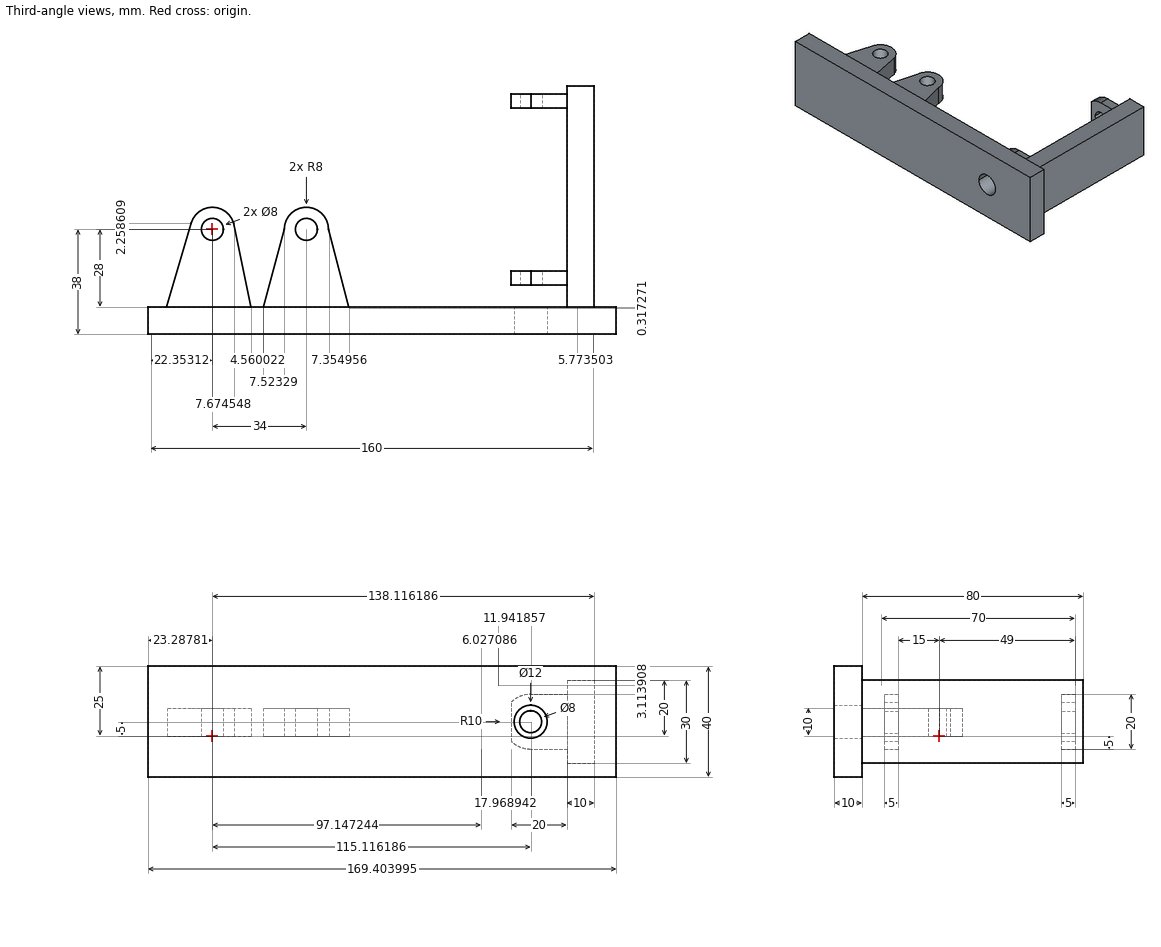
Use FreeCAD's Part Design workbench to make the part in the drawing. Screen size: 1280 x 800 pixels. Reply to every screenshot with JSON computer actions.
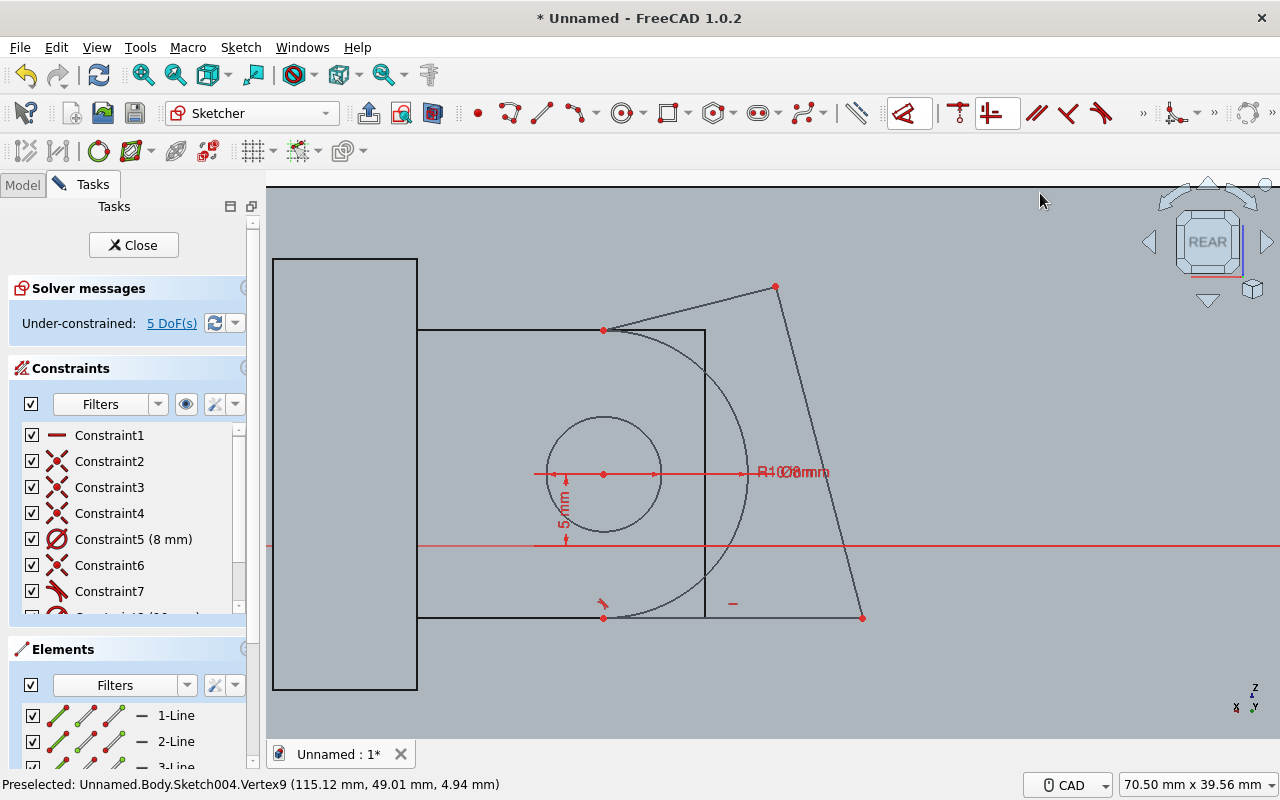
{"action": "left_click", "coordinate": [682, 618]}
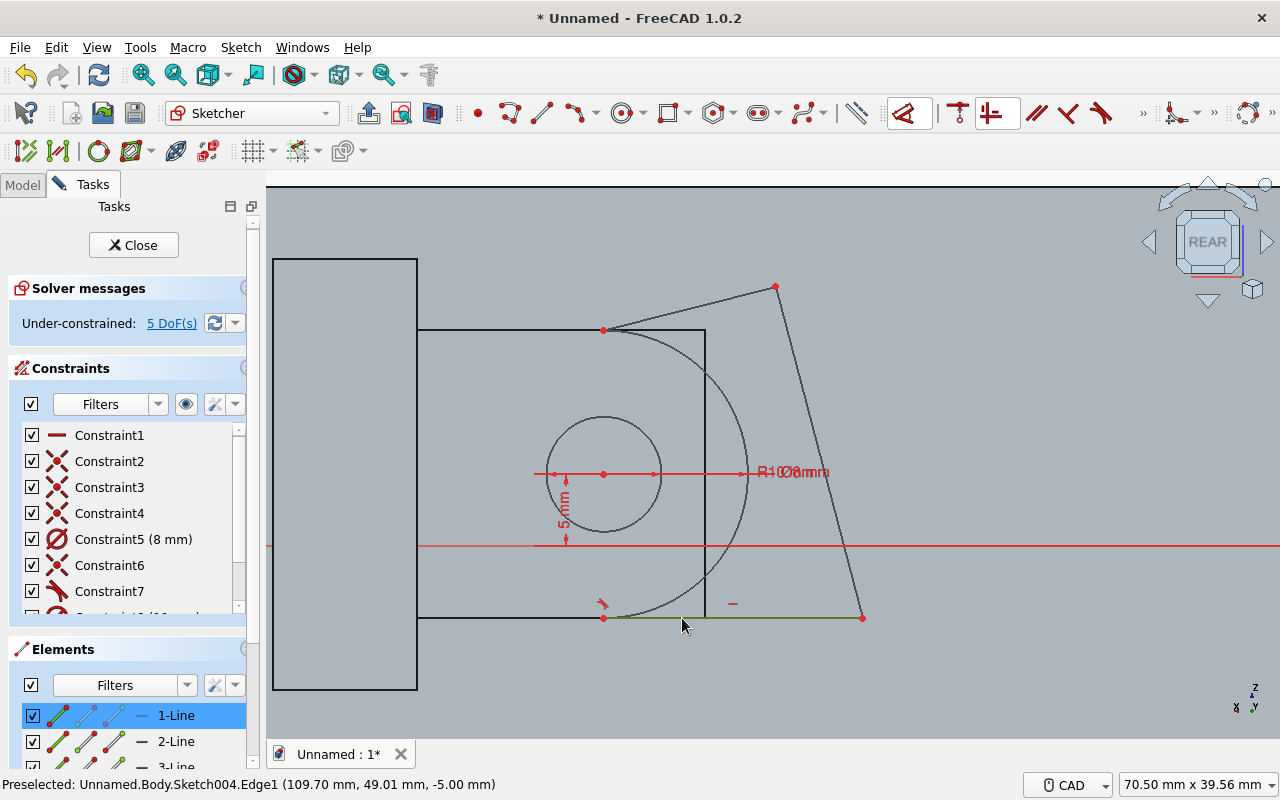
{"action": "left_click", "coordinate": [926, 114]}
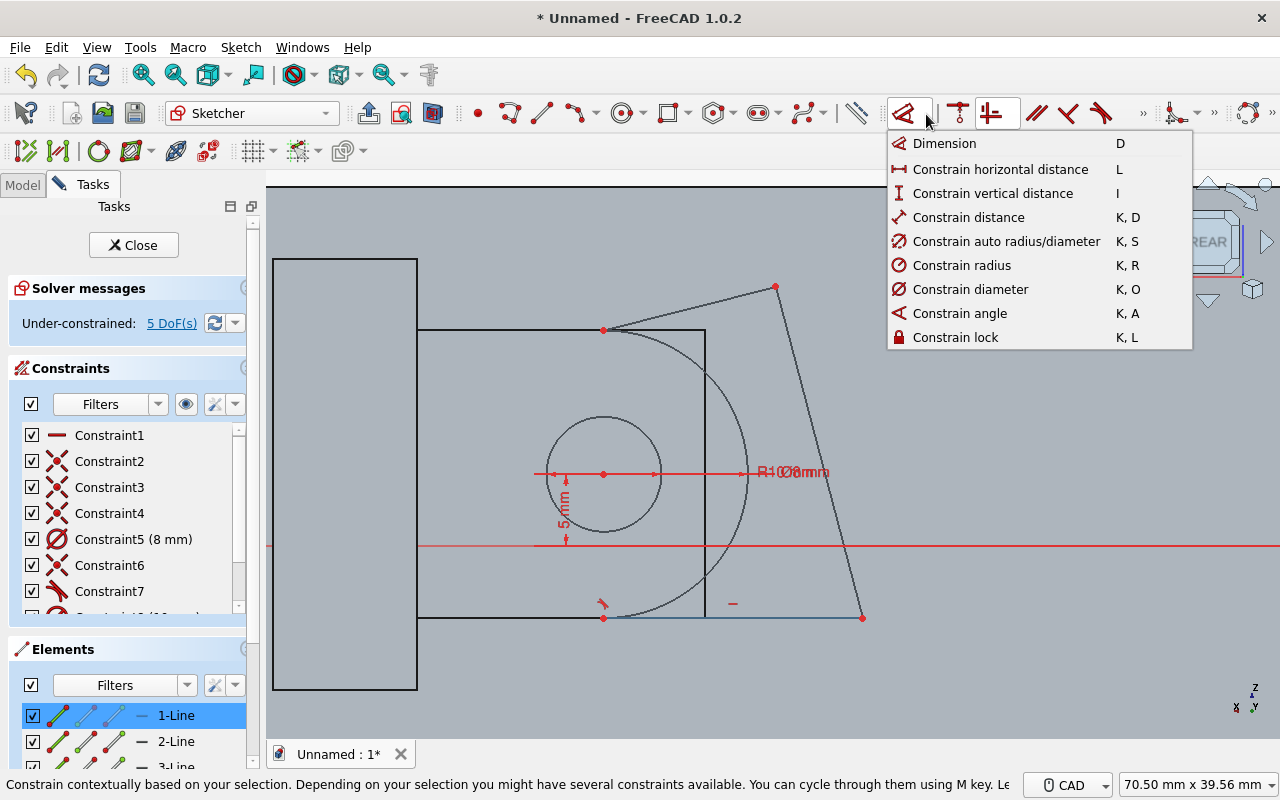
{"action": "left_click", "coordinate": [1040, 169]}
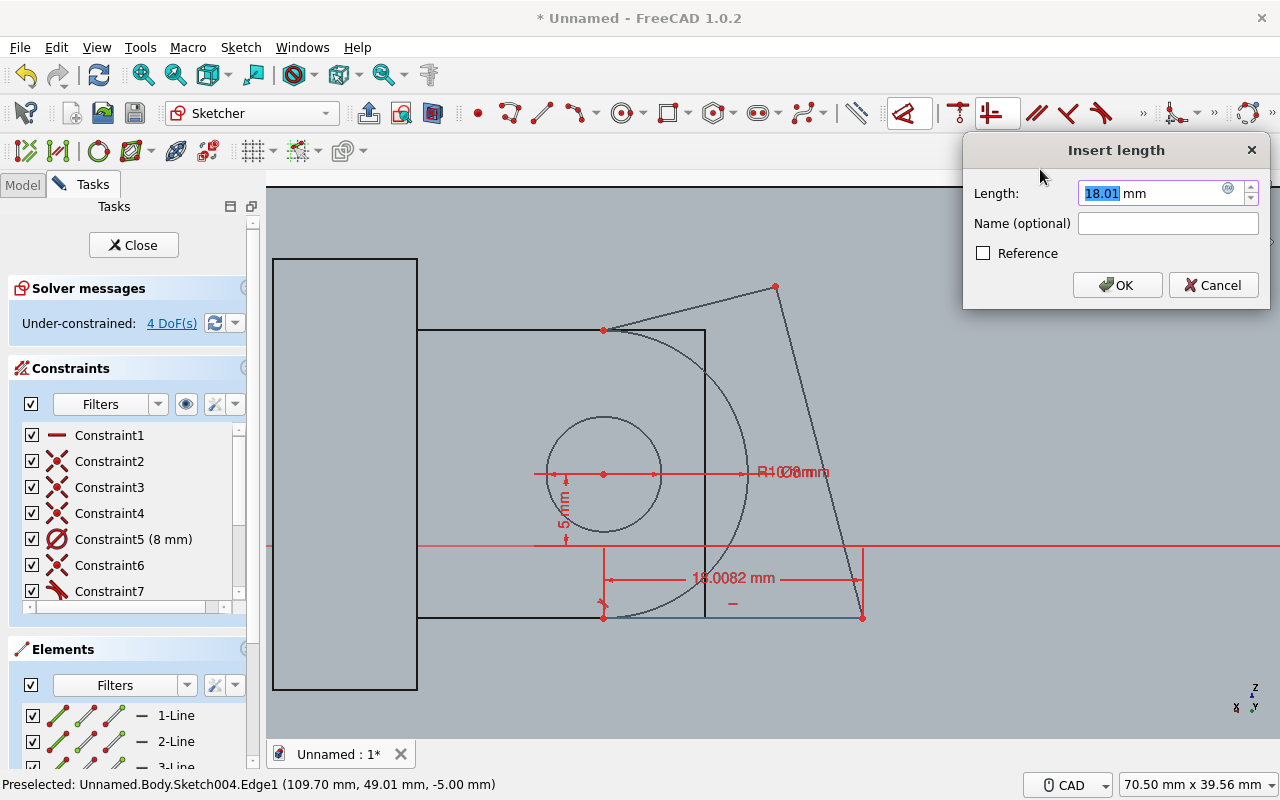
{"action": "type", "text": "17.968942"}
{"action": "key", "text": "Return"}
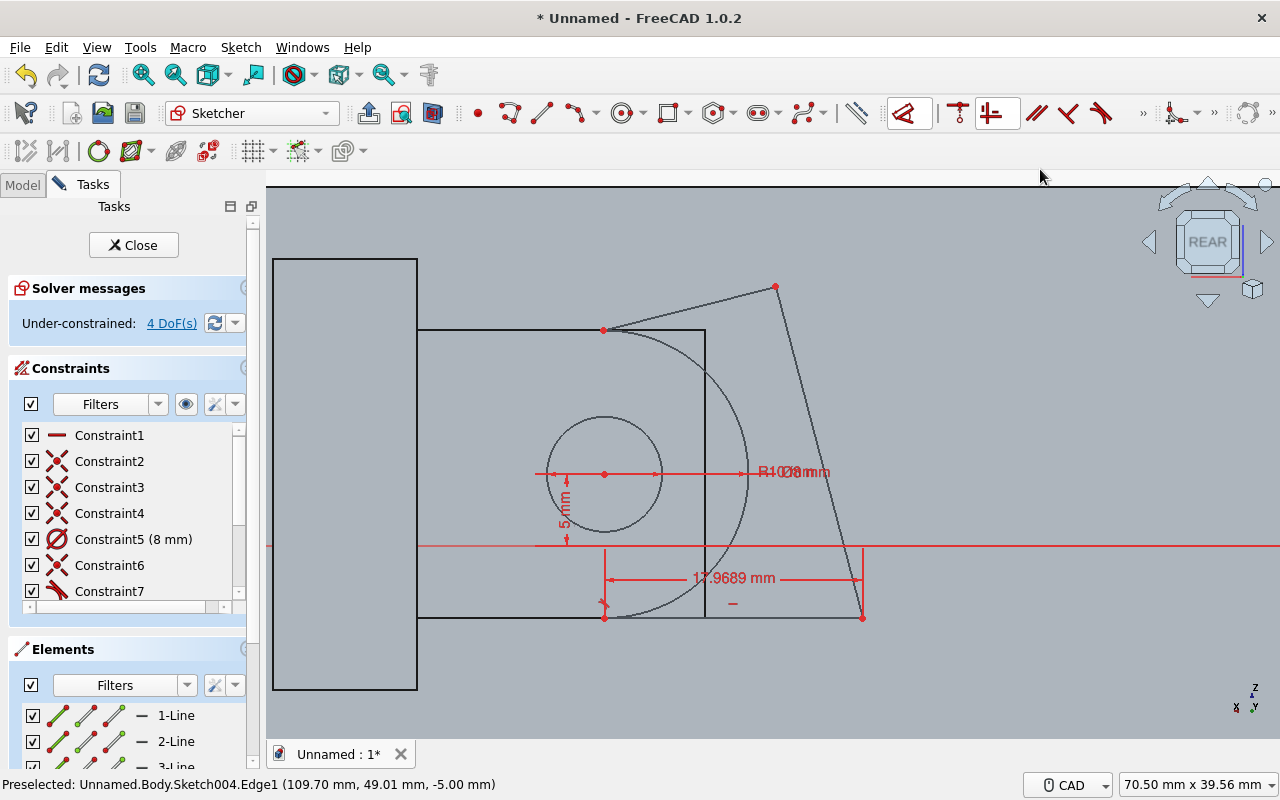
{"action": "left_click", "coordinate": [837, 519]}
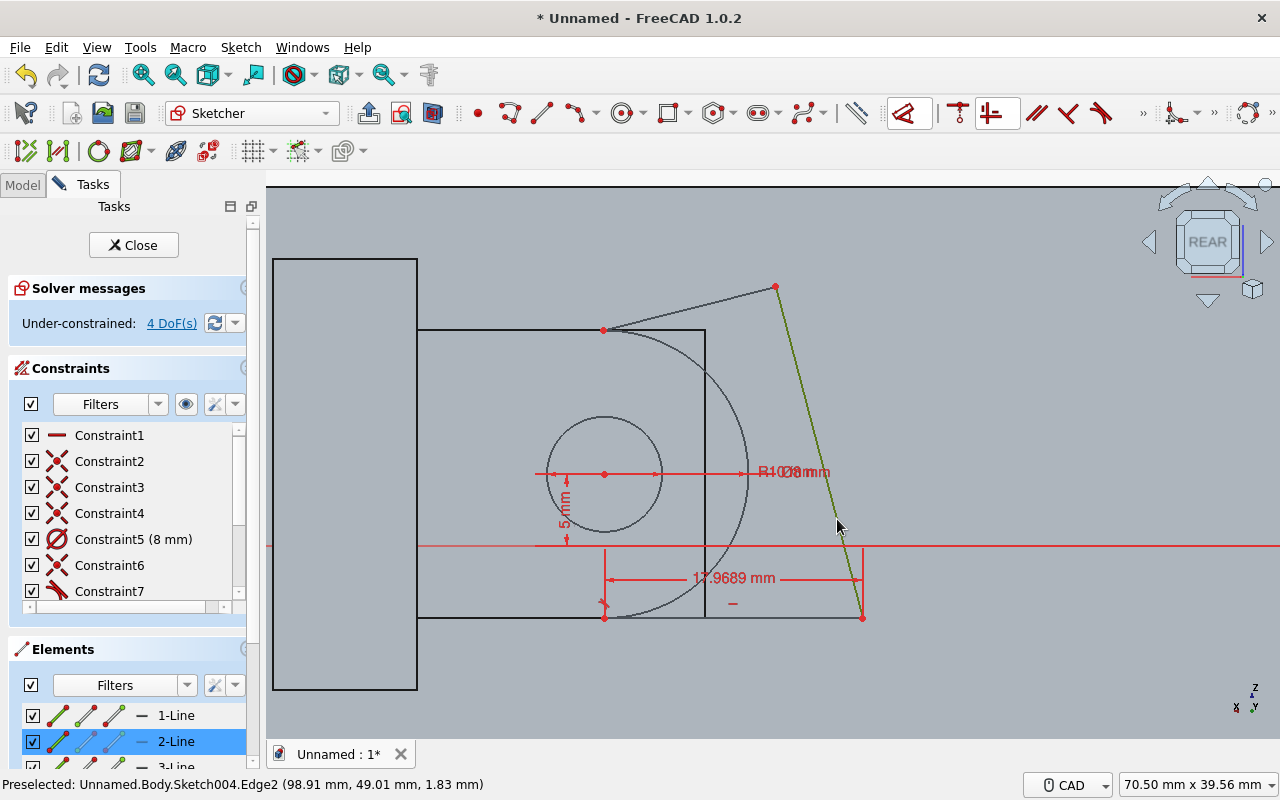
{"action": "key", "text": "l"}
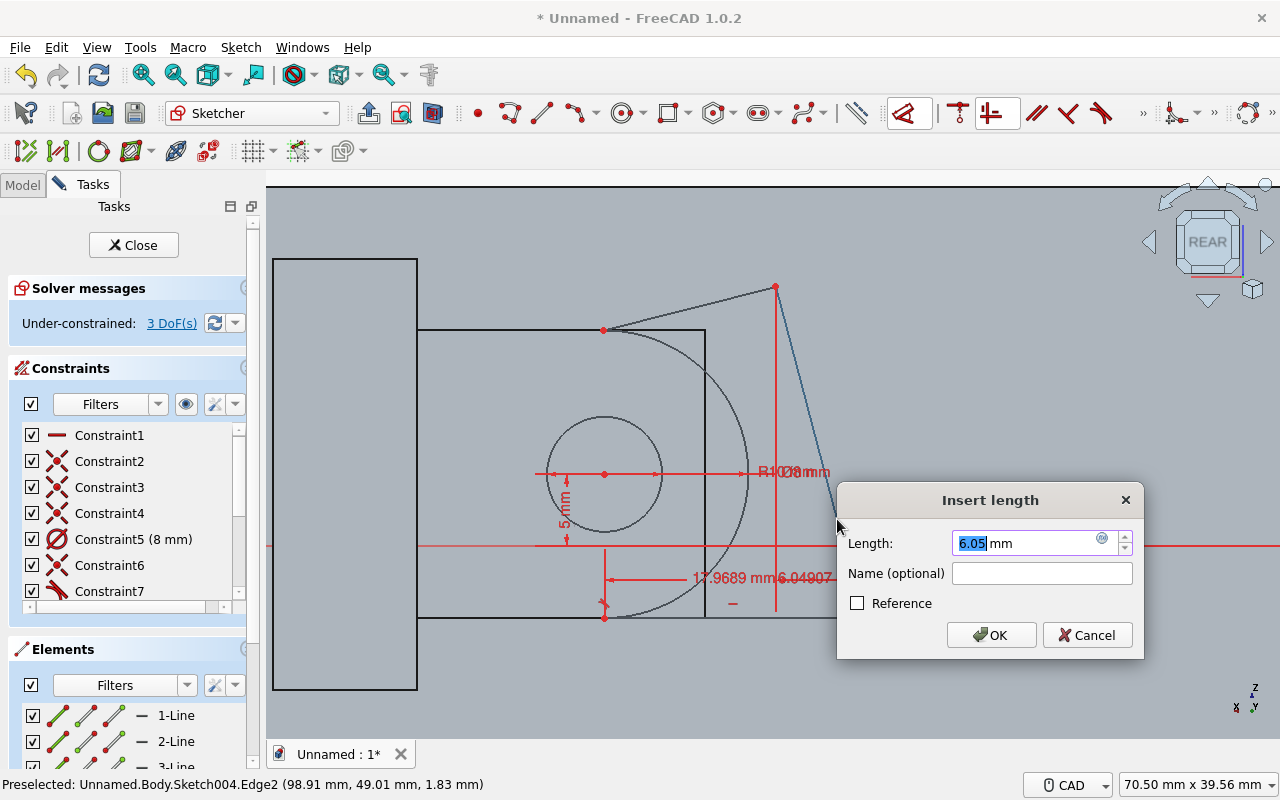
{"action": "type", "text": "6.027086"}
{"action": "key", "text": "Return"}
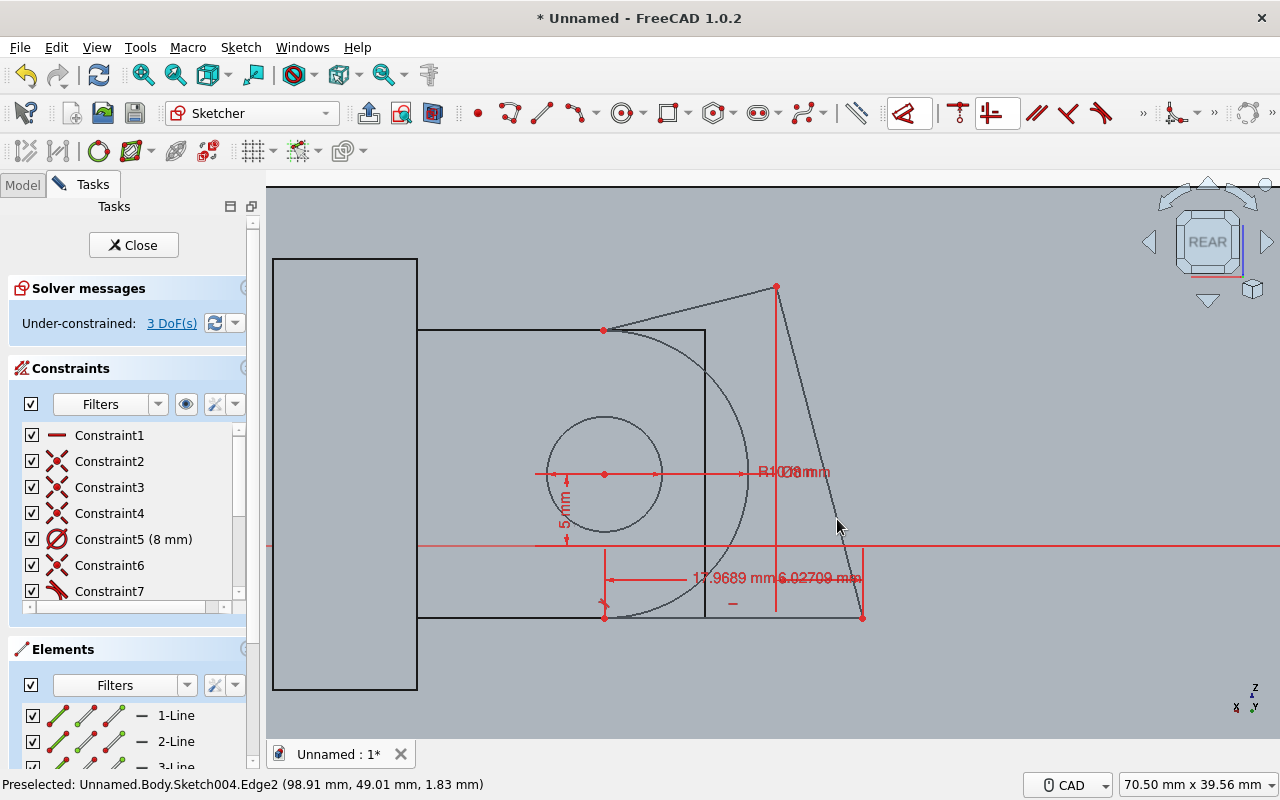
{"action": "left_click", "coordinate": [725, 300]}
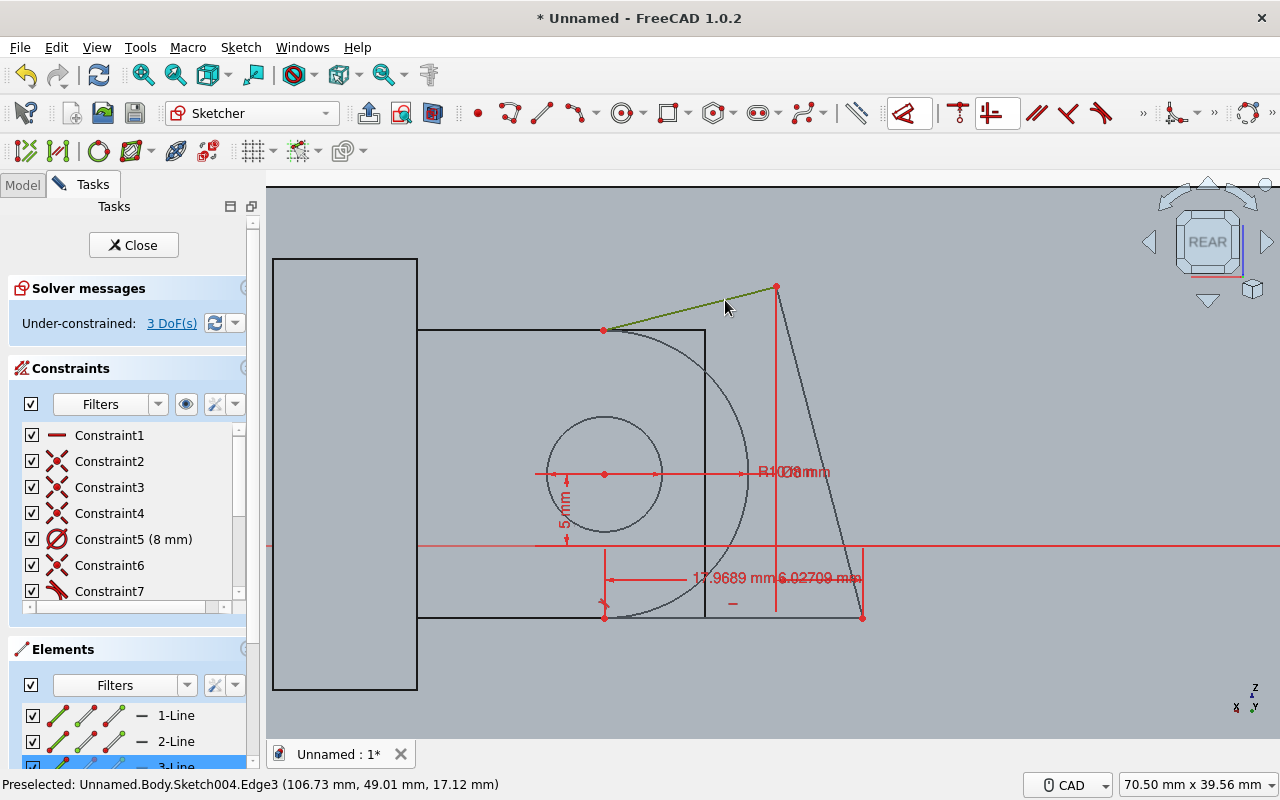
{"action": "key", "text": "i"}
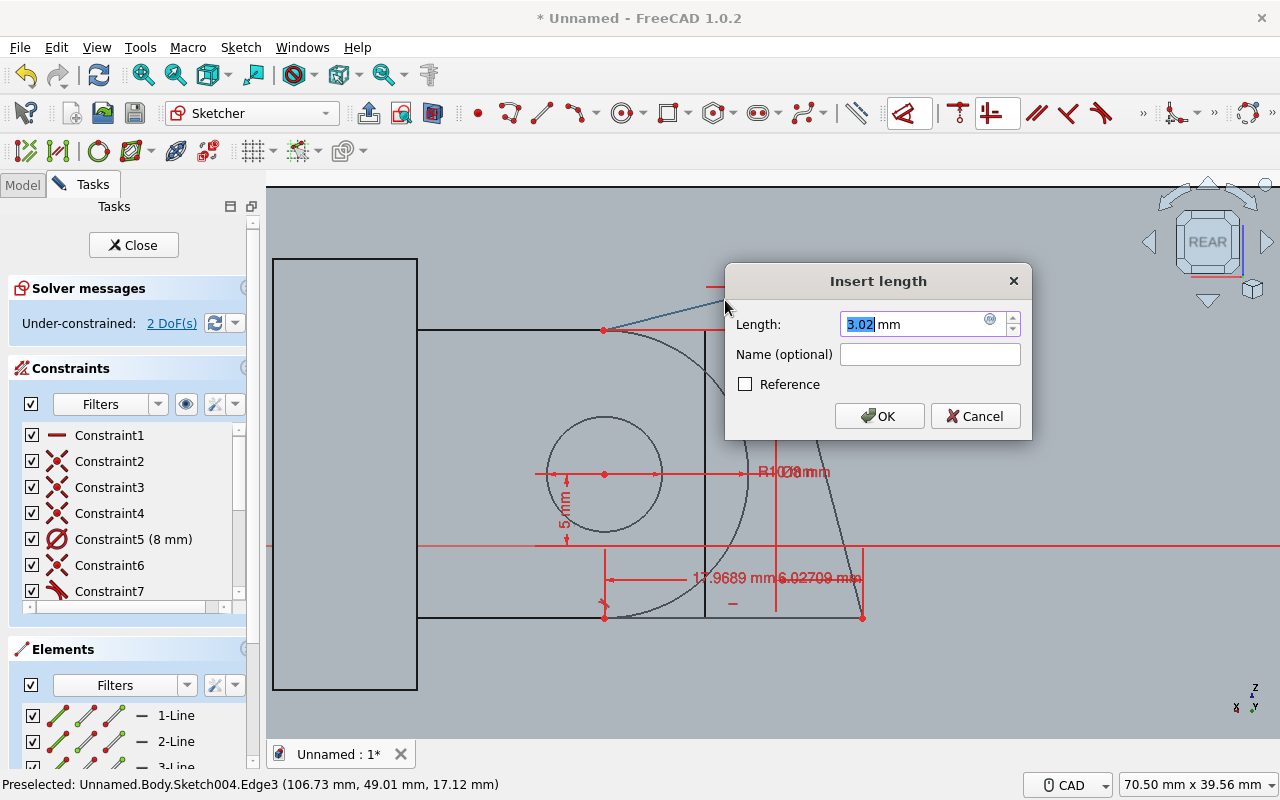
{"action": "type", "text": "3.113908"}
{"action": "key", "text": "Return"}